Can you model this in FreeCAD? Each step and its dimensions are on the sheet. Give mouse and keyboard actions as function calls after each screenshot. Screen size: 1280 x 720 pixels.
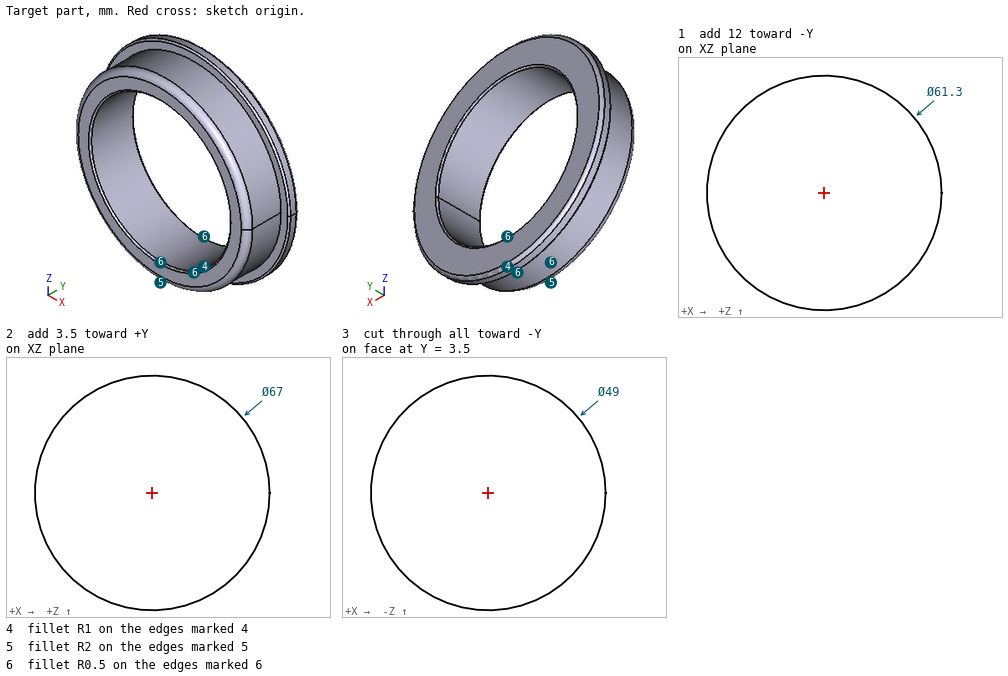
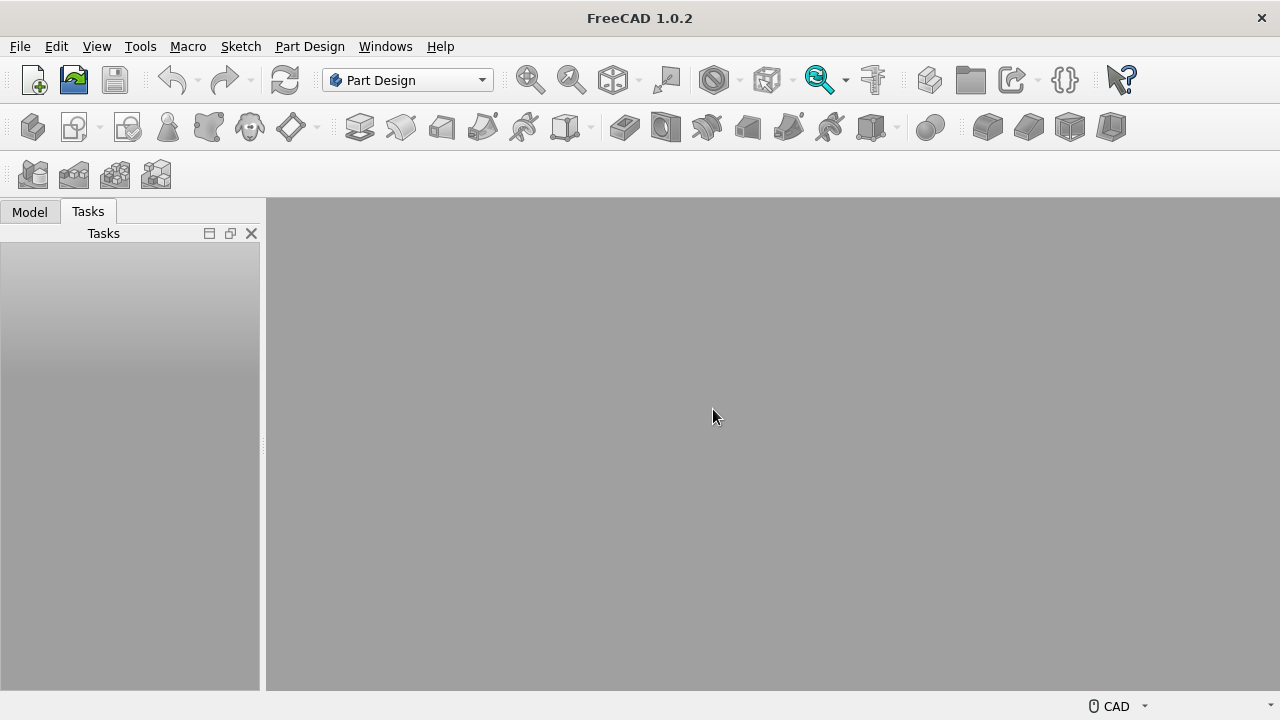
click(33, 80)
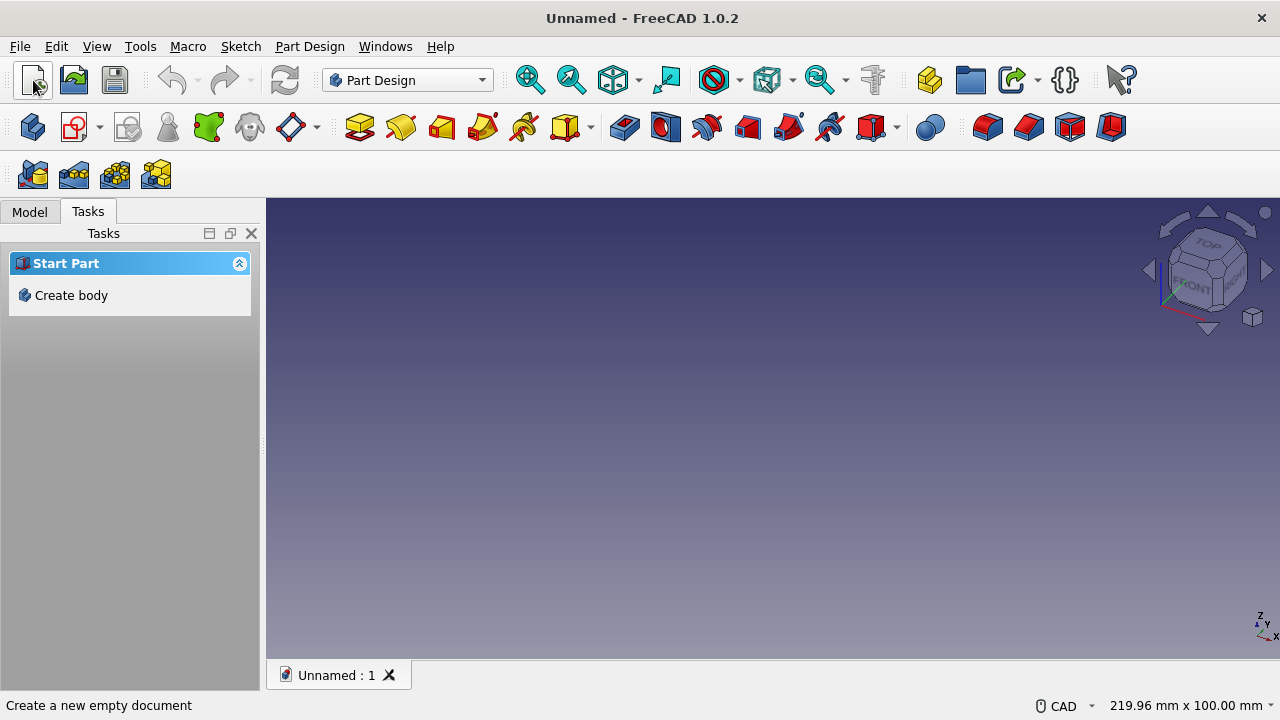
click(74, 128)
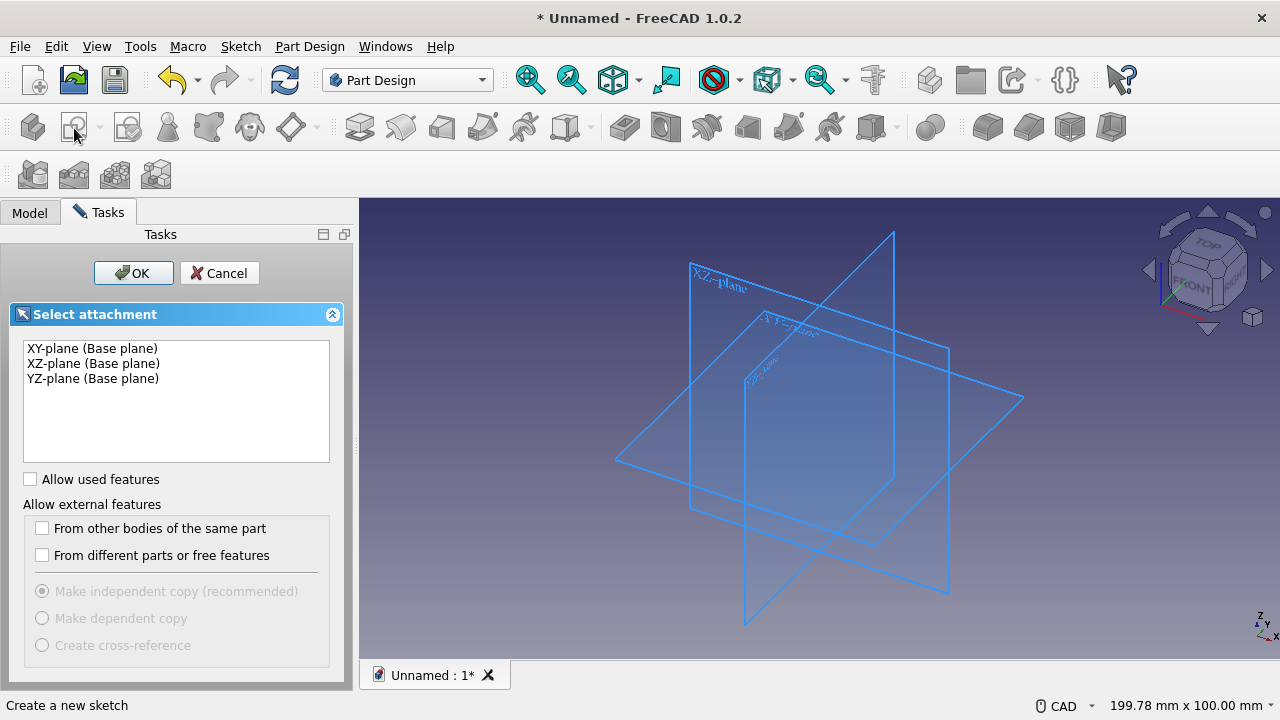
click(84, 364)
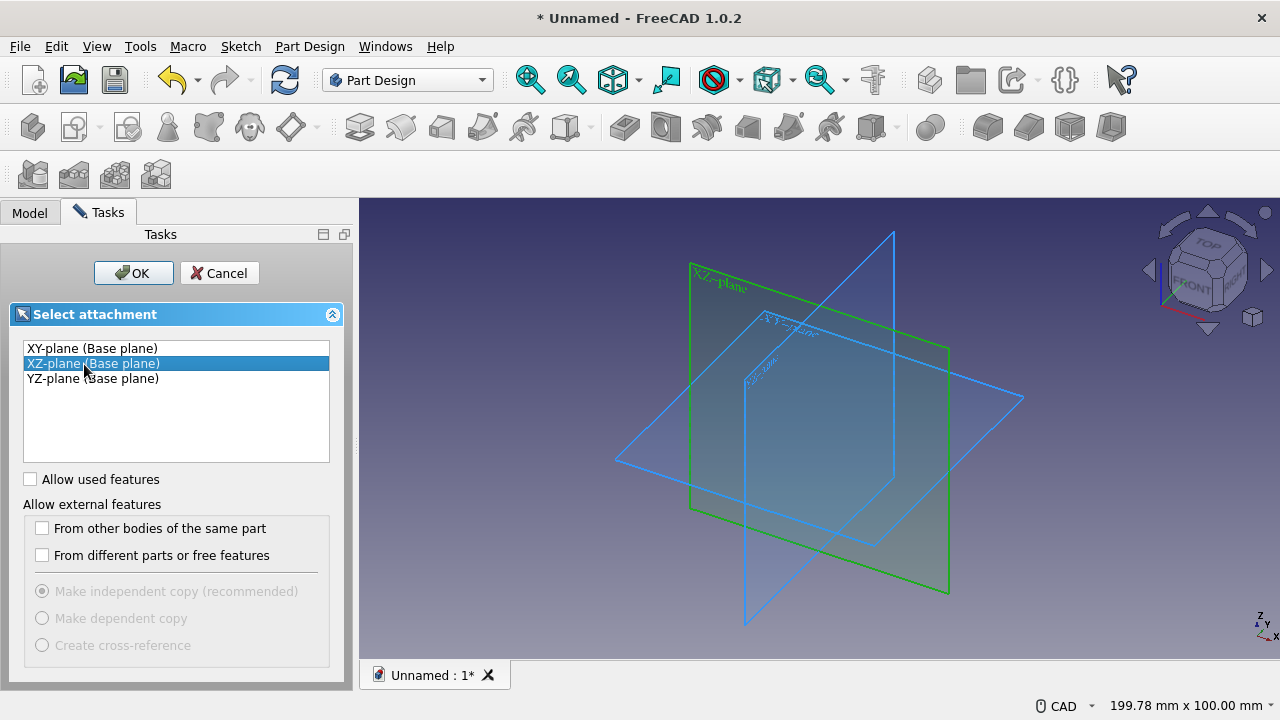
click(134, 273)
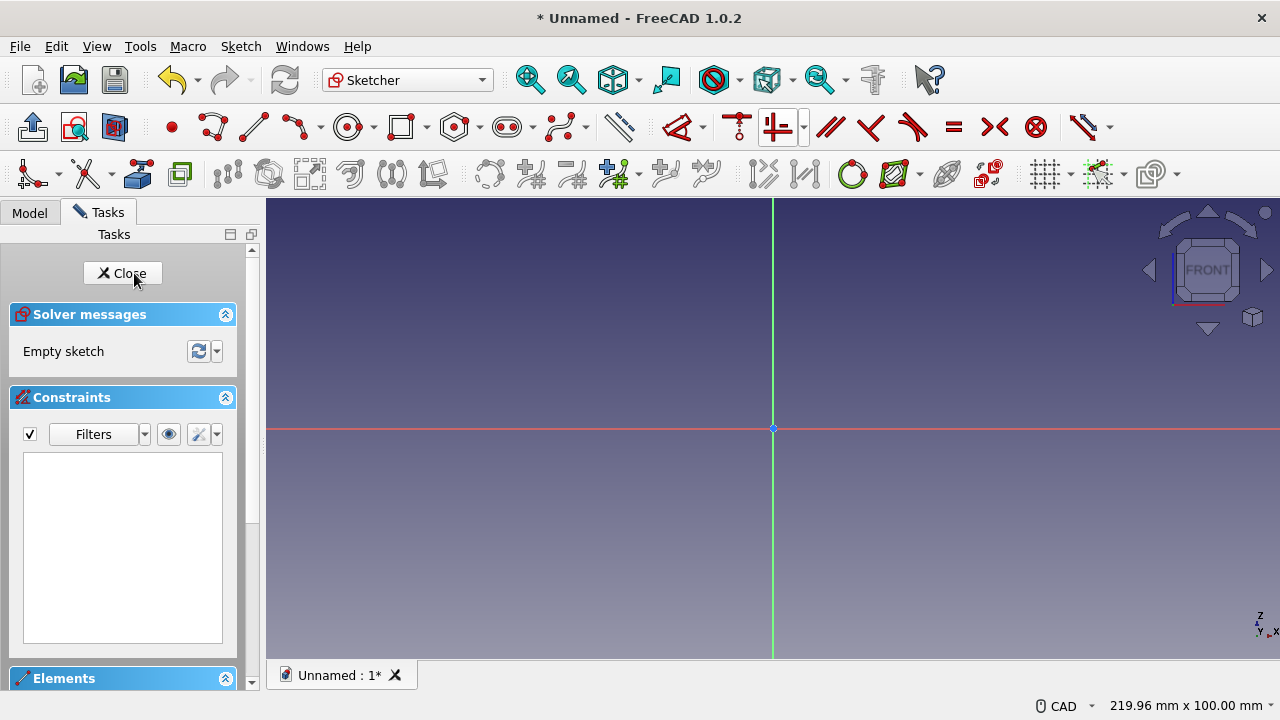
click(348, 128)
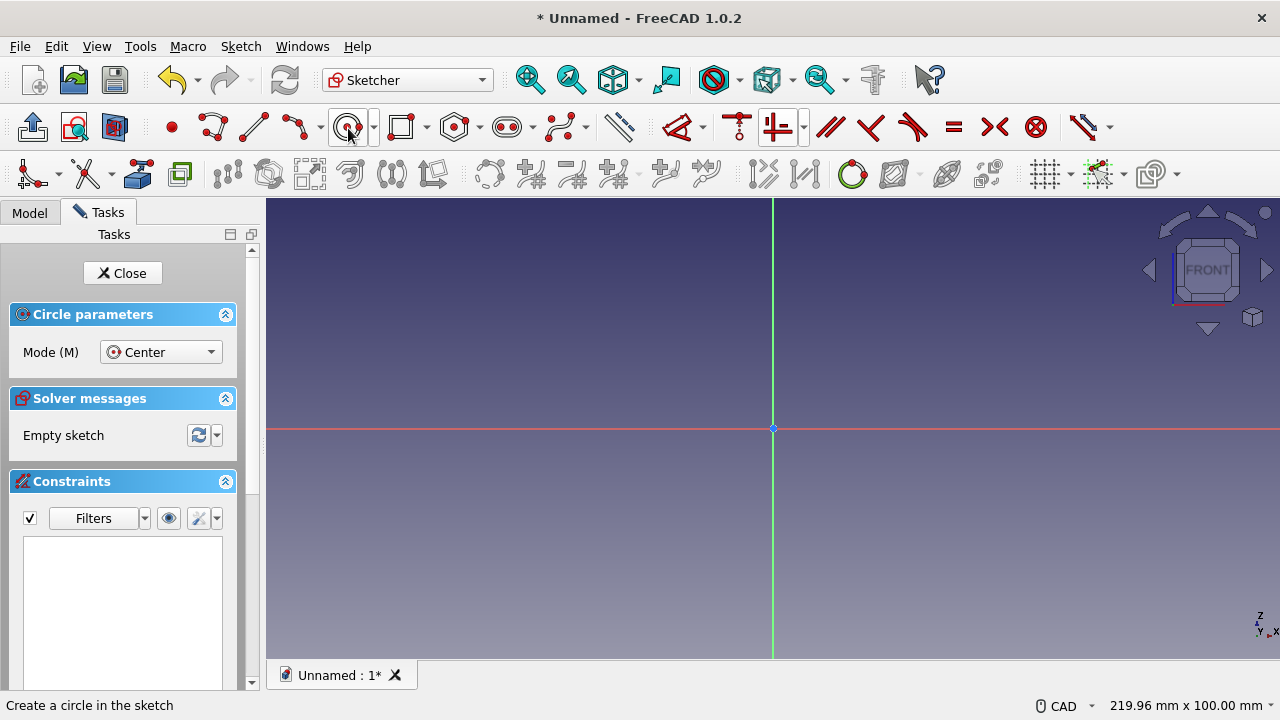
click(773, 428)
click(873, 329)
key(Escape)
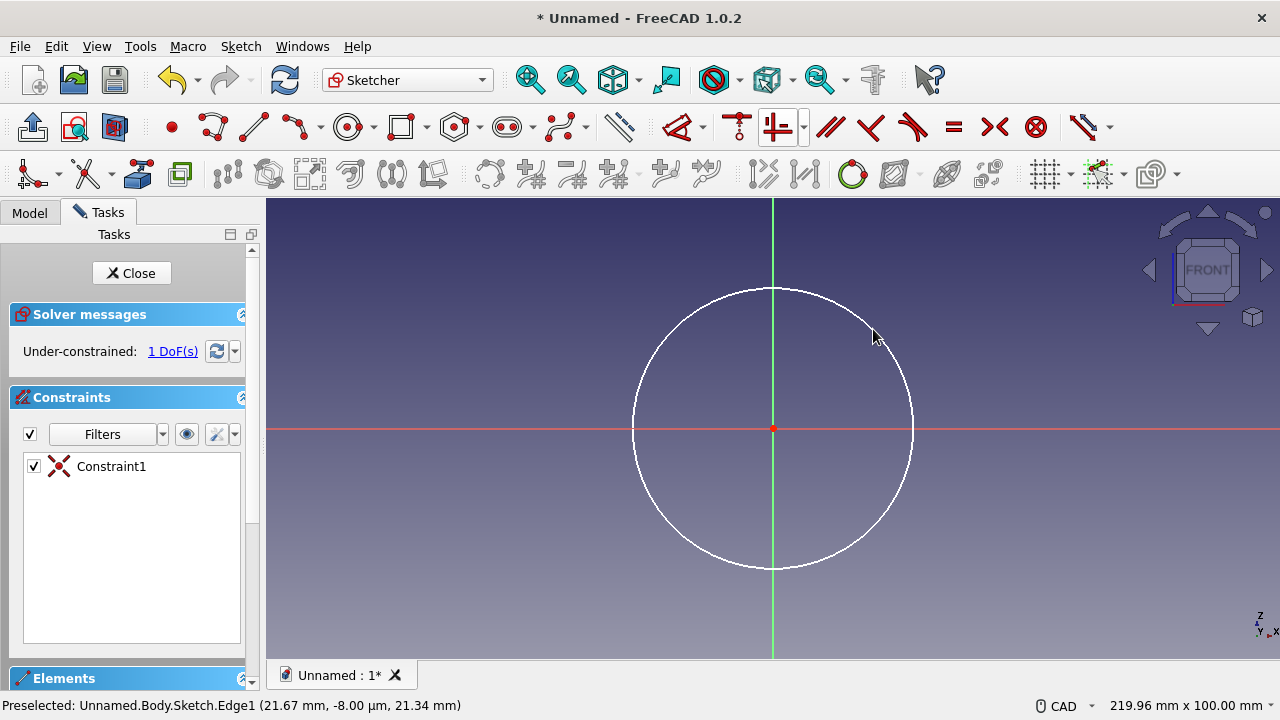
click(676, 128)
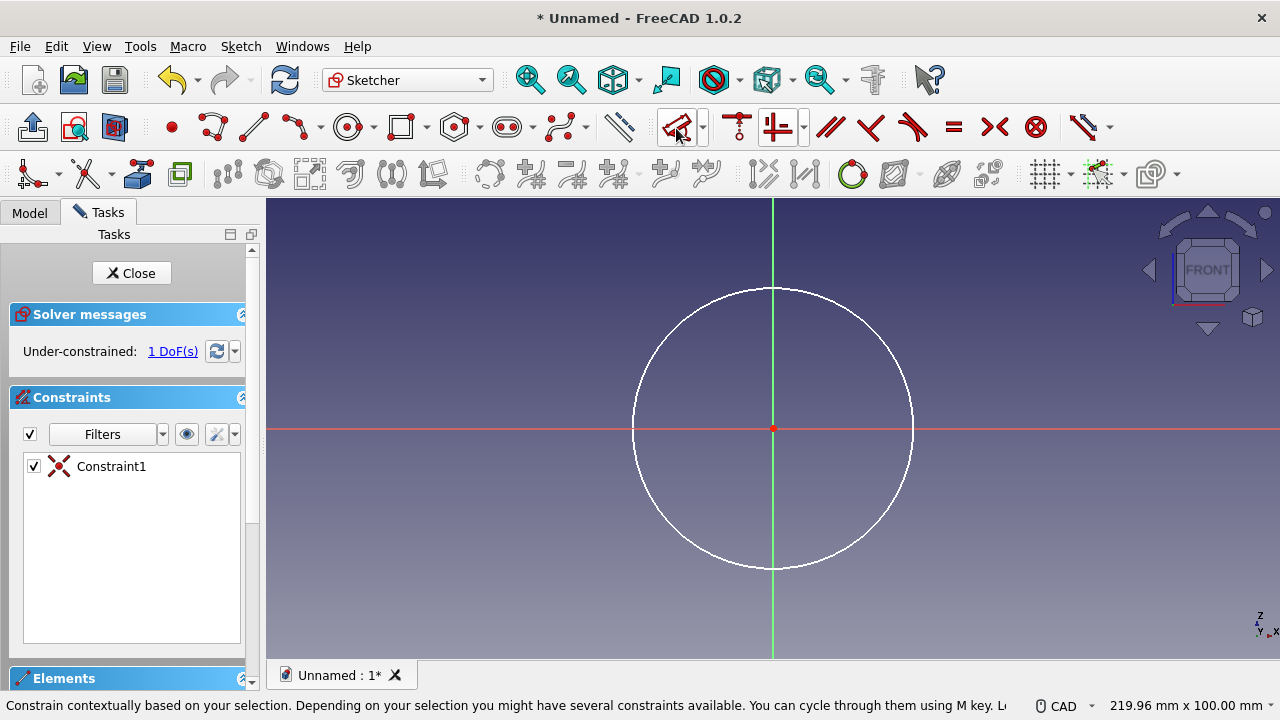
click(872, 329)
click(895, 306)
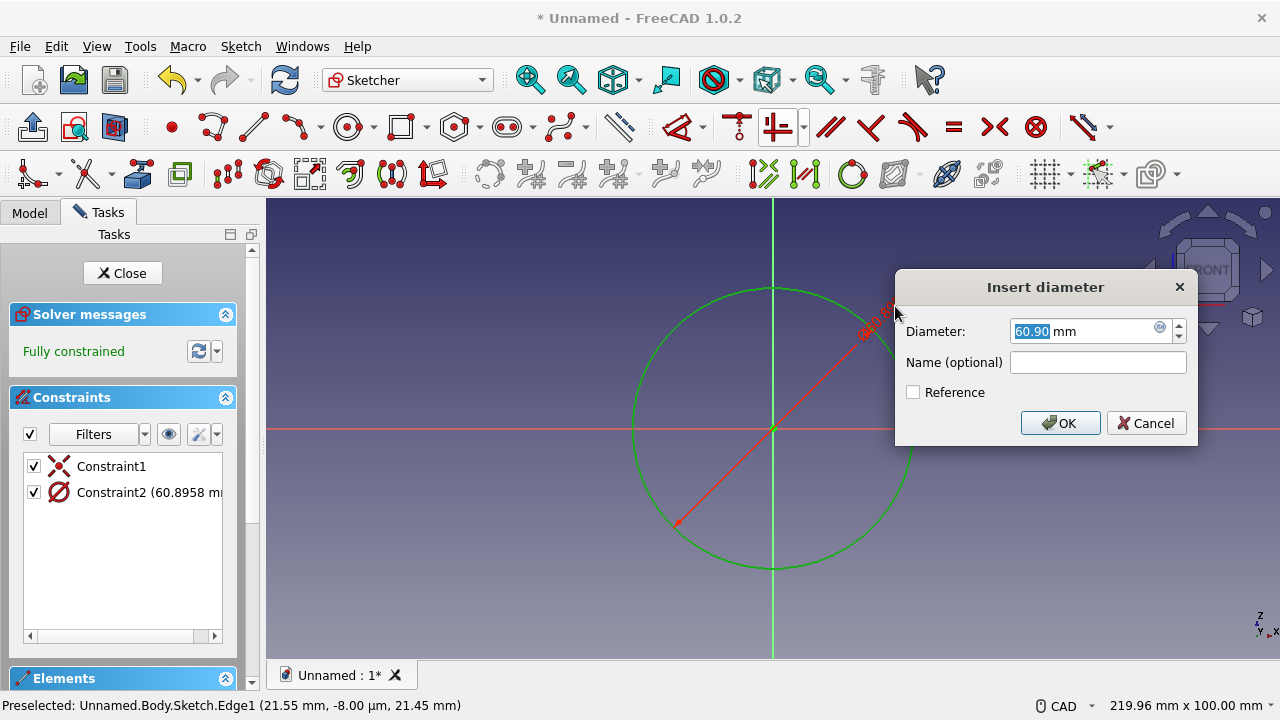
text(61.3)
key(Return)
key(Escape)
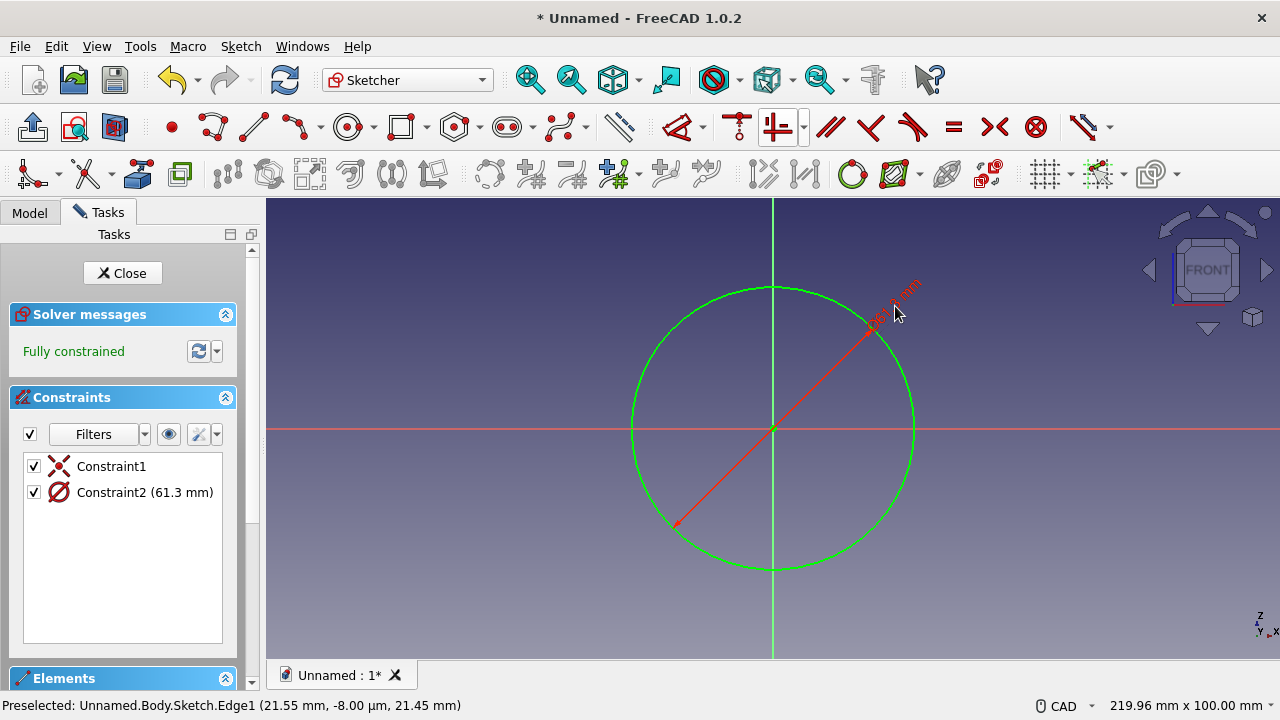
click(123, 273)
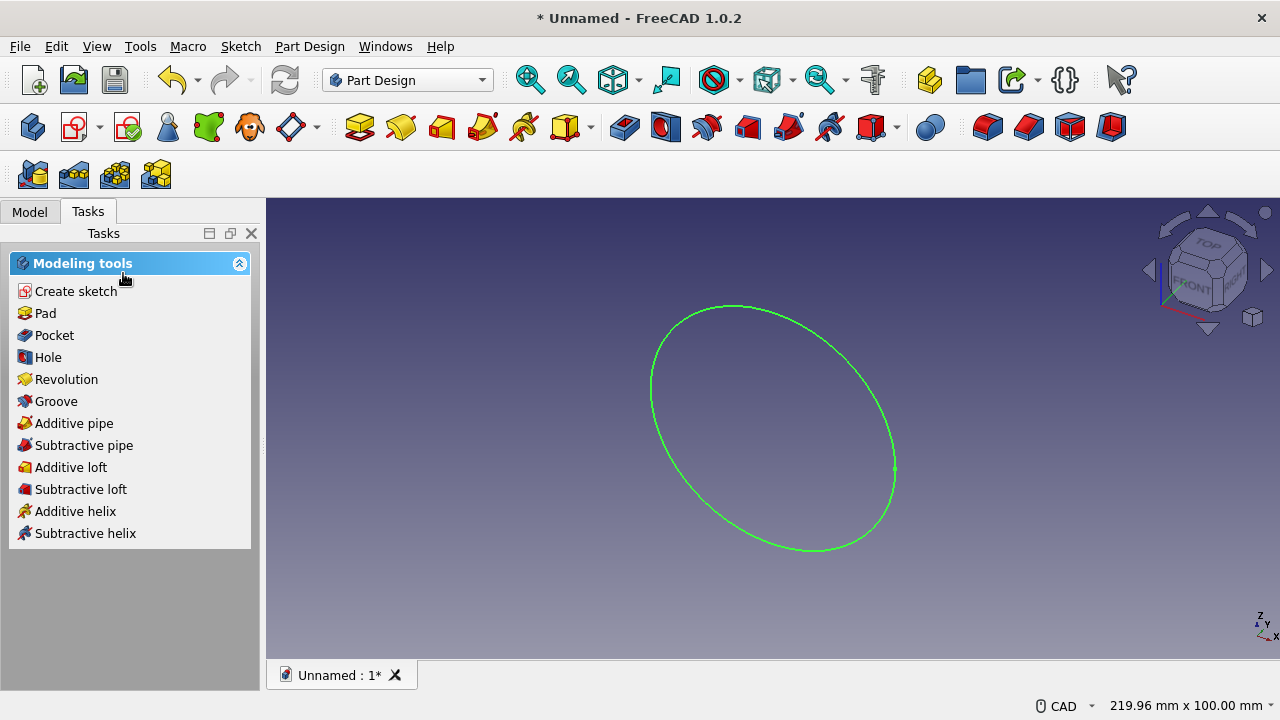
click(360, 128)